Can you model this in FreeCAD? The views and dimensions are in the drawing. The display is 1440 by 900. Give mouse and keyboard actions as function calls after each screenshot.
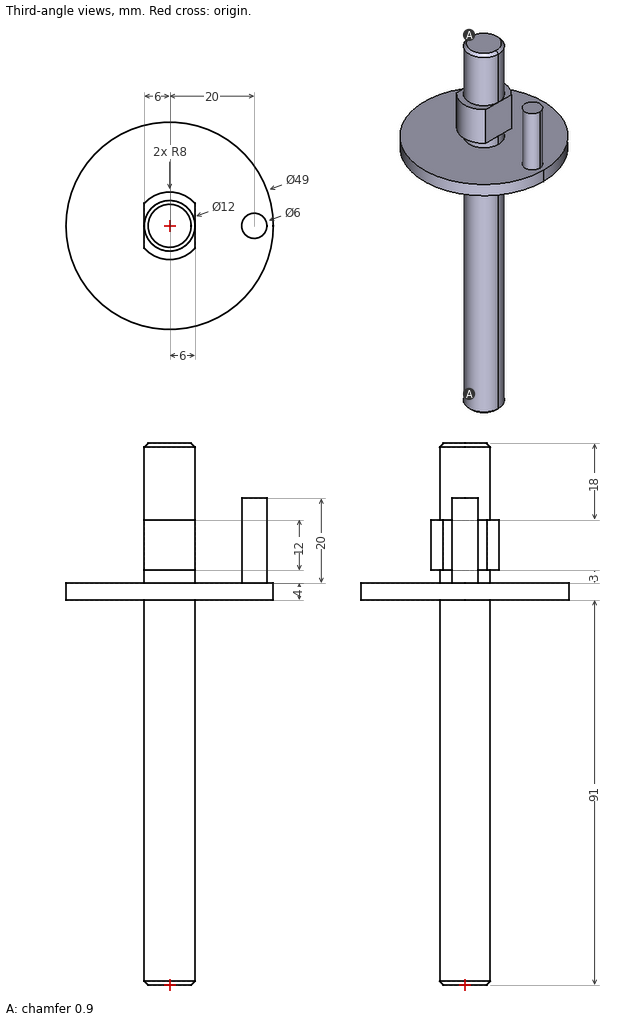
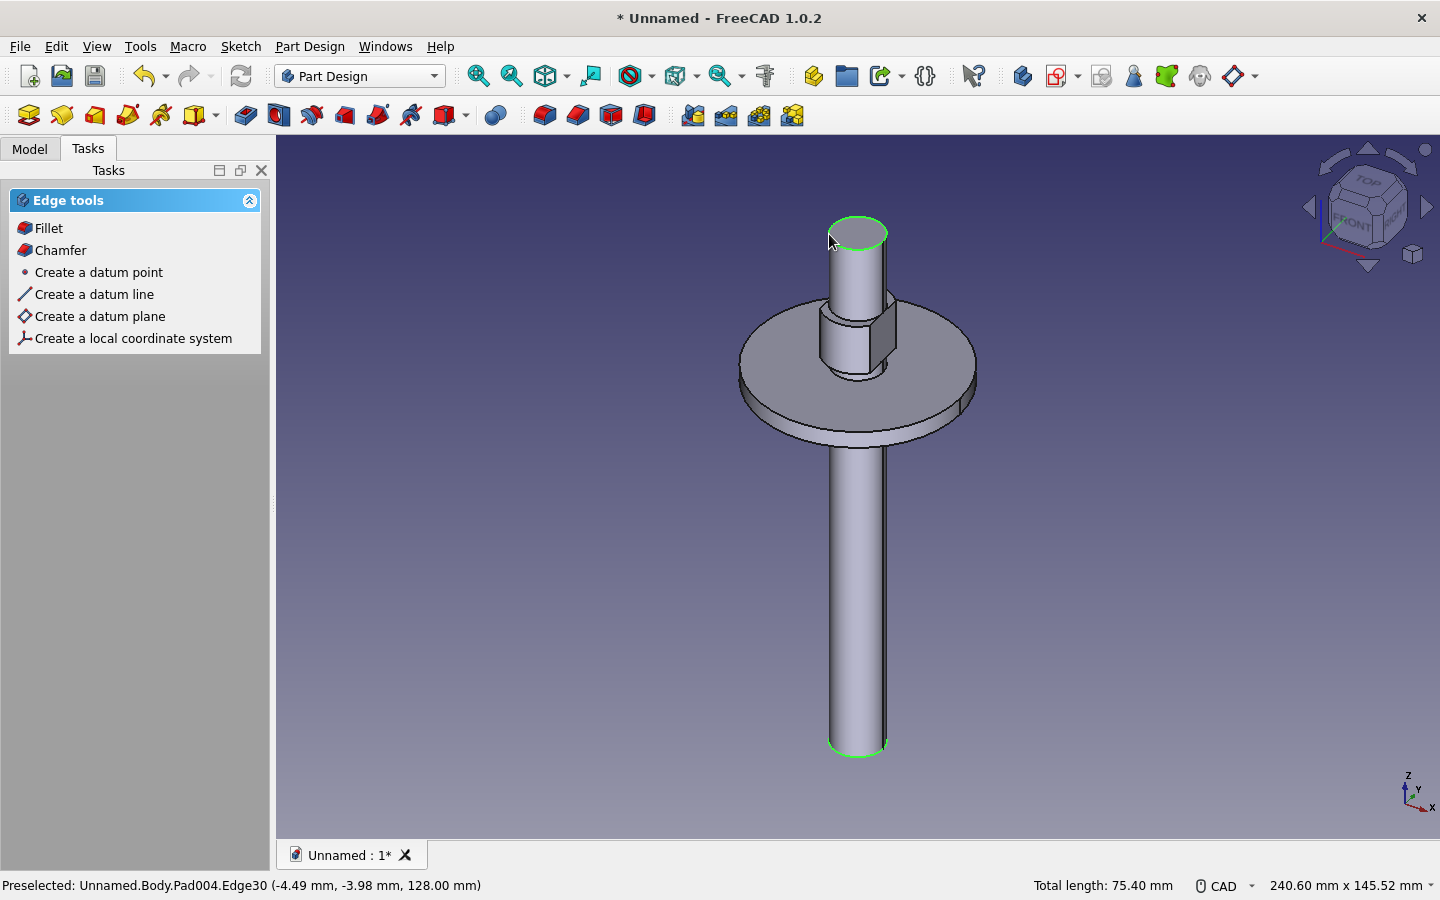
click(578, 116)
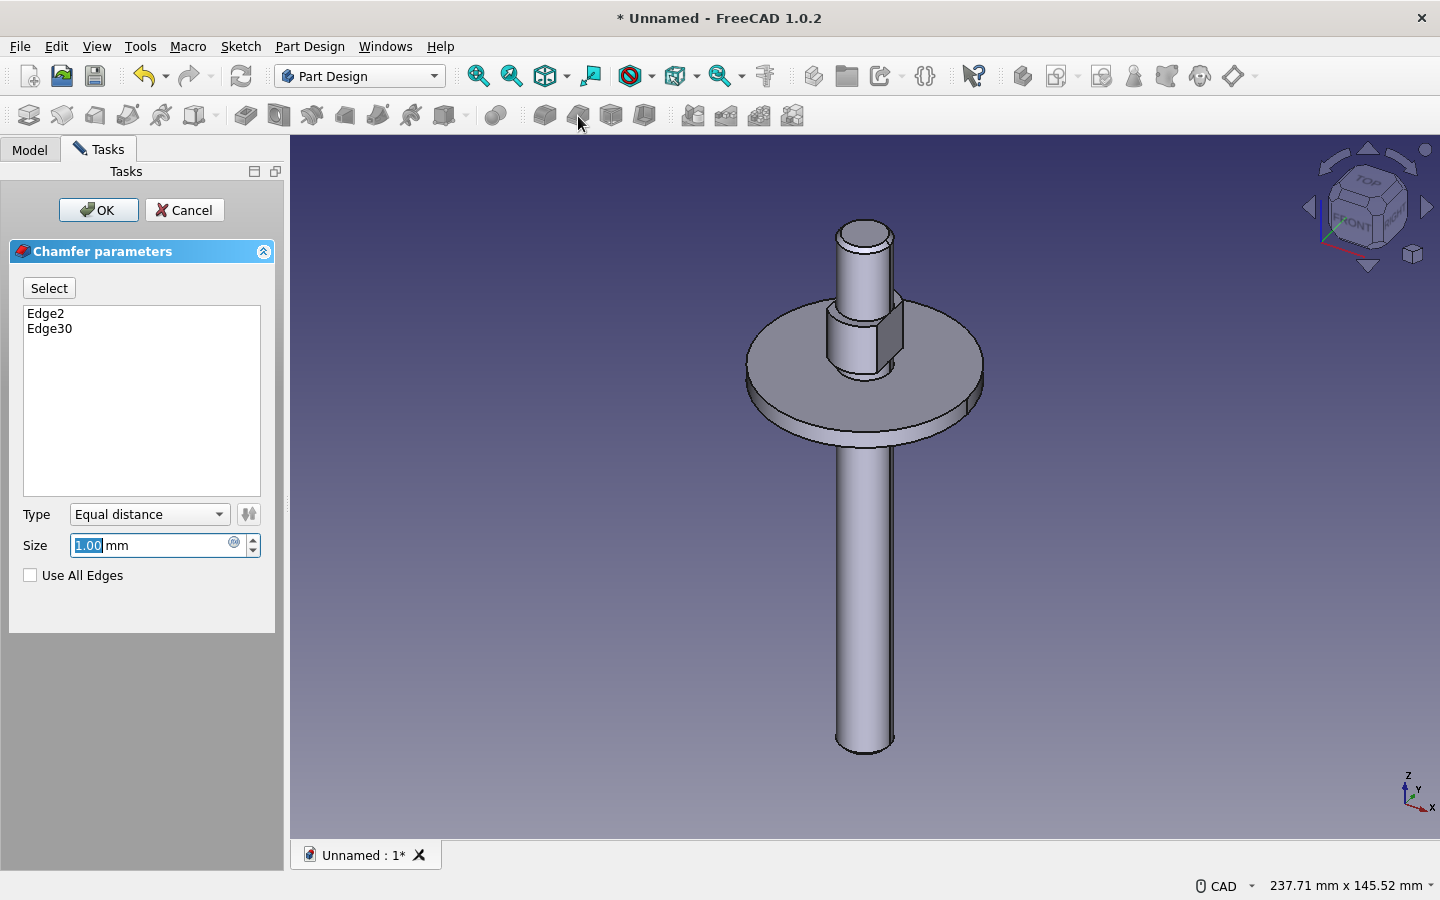
text(0.9)
key(Tab)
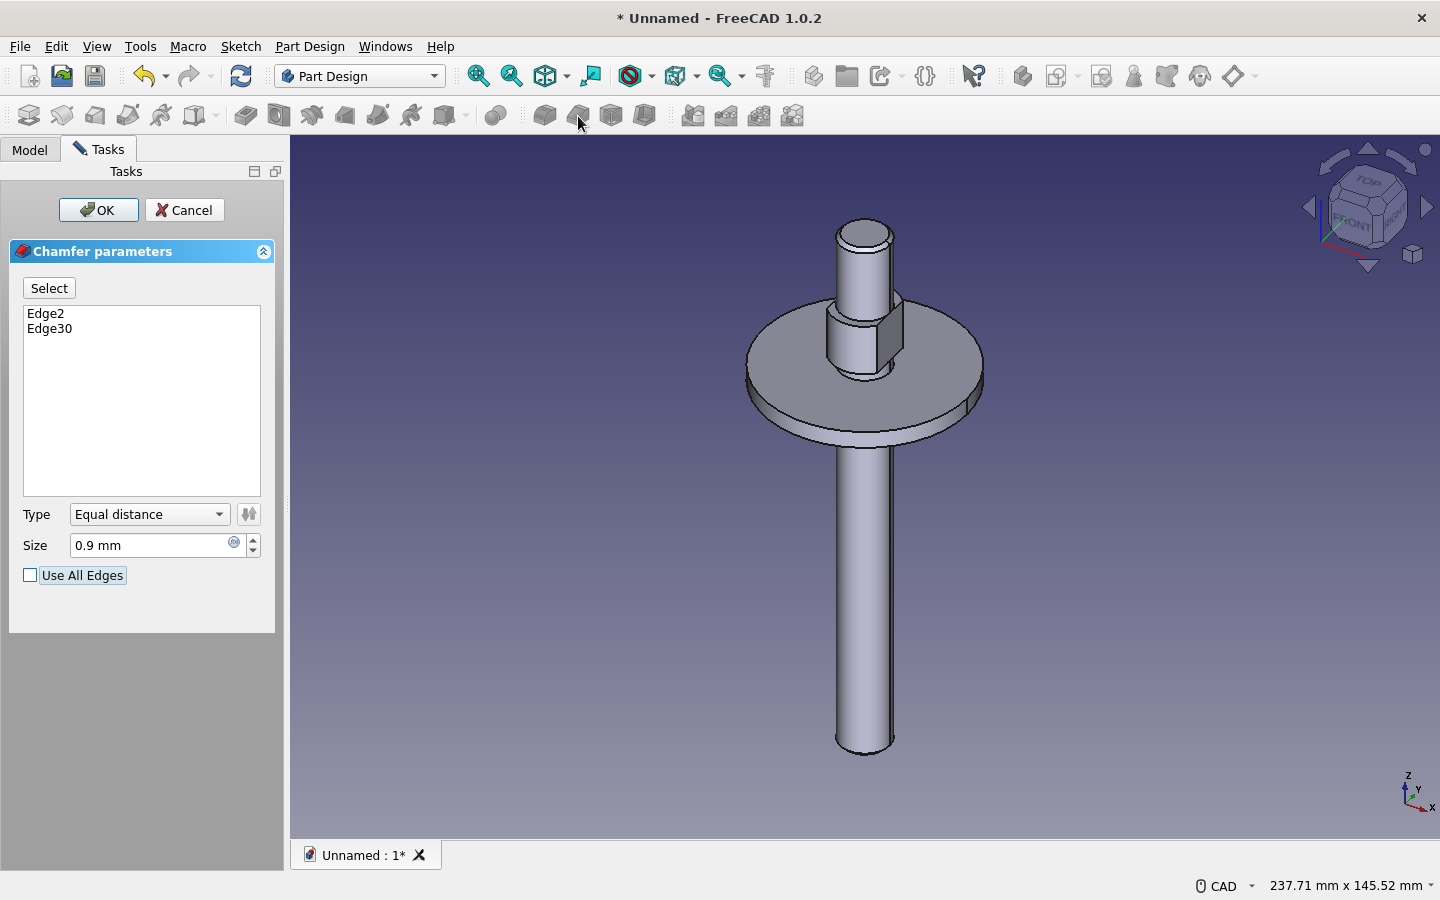
click(99, 210)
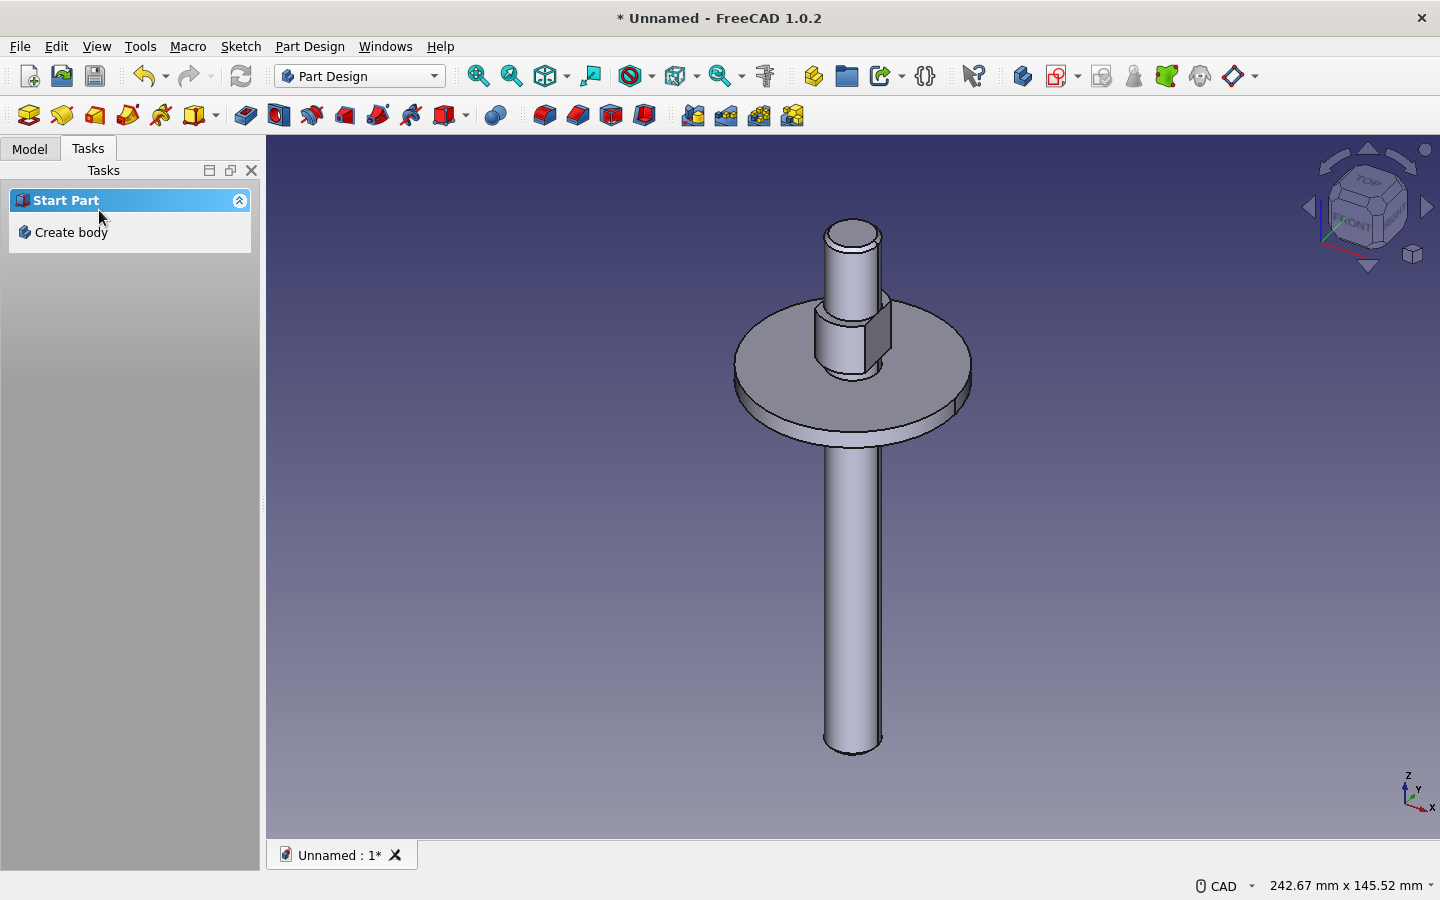
click(928, 366)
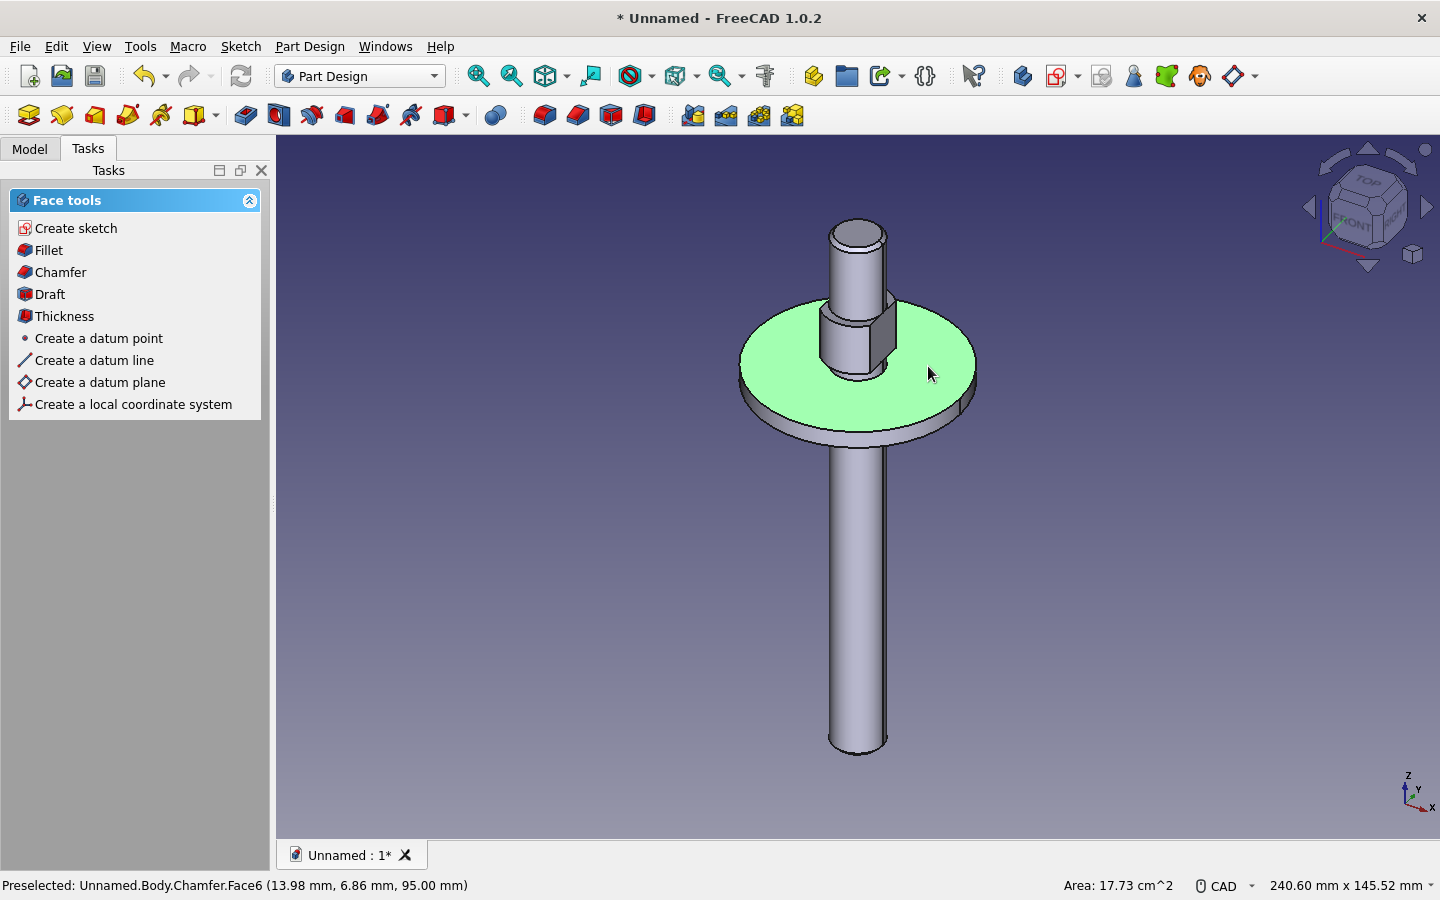
click(1056, 76)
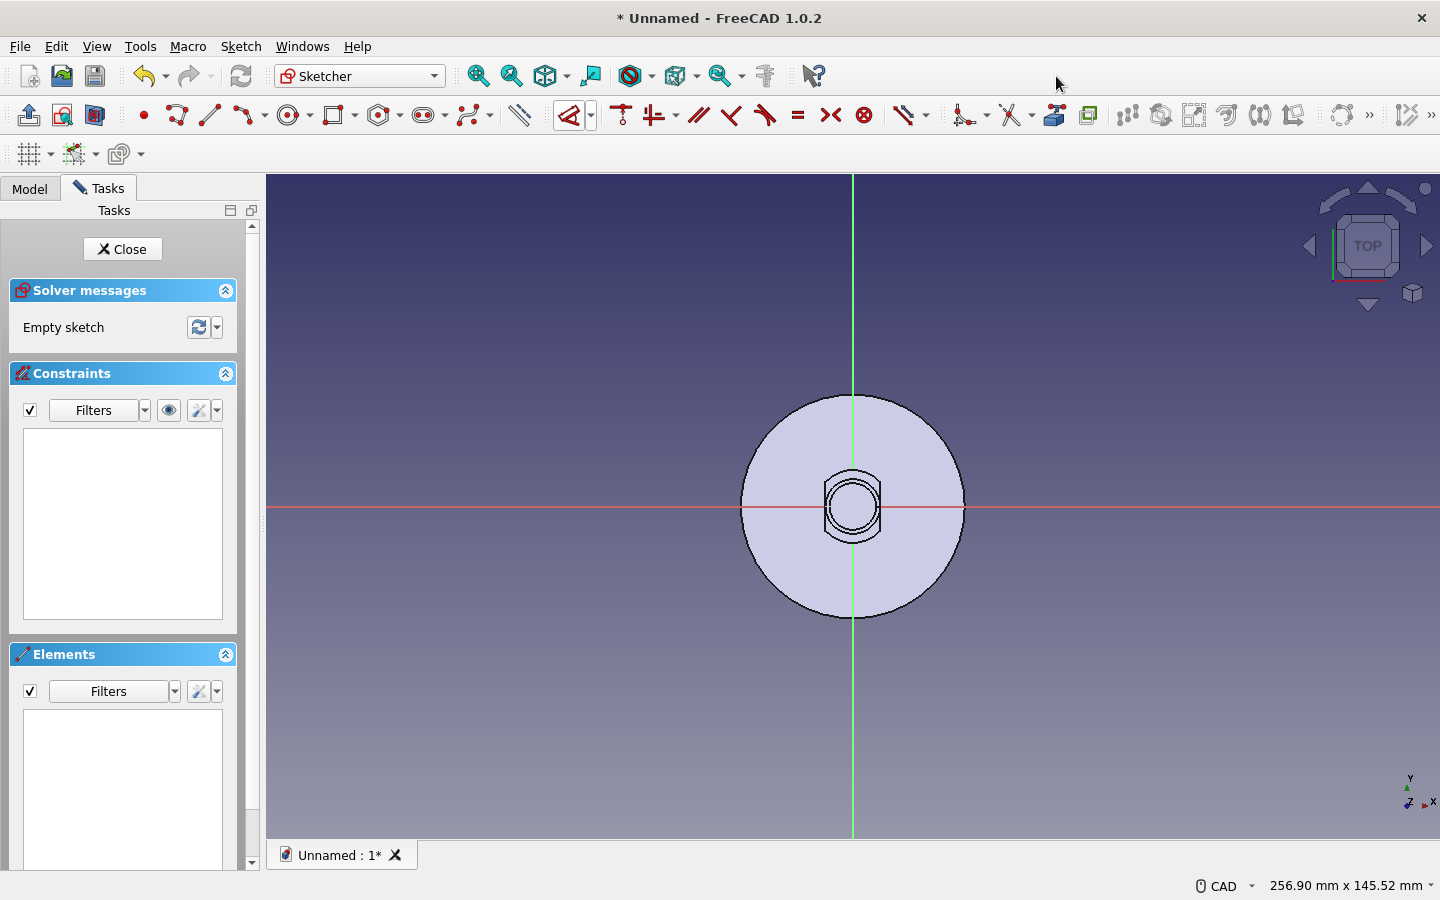
key(q)
key(s)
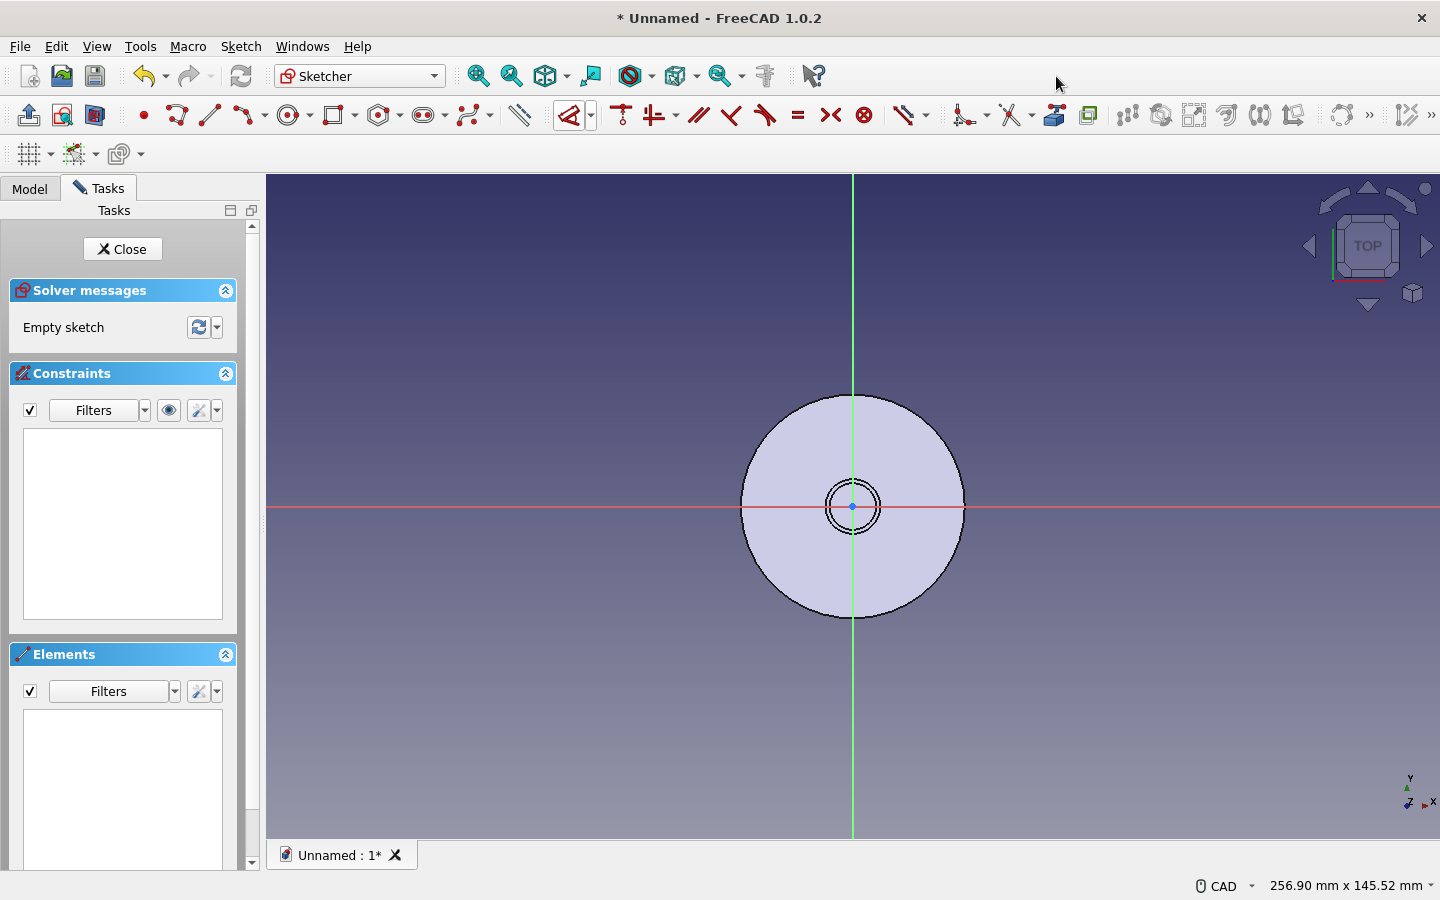
scroll(955, 506, up, 14)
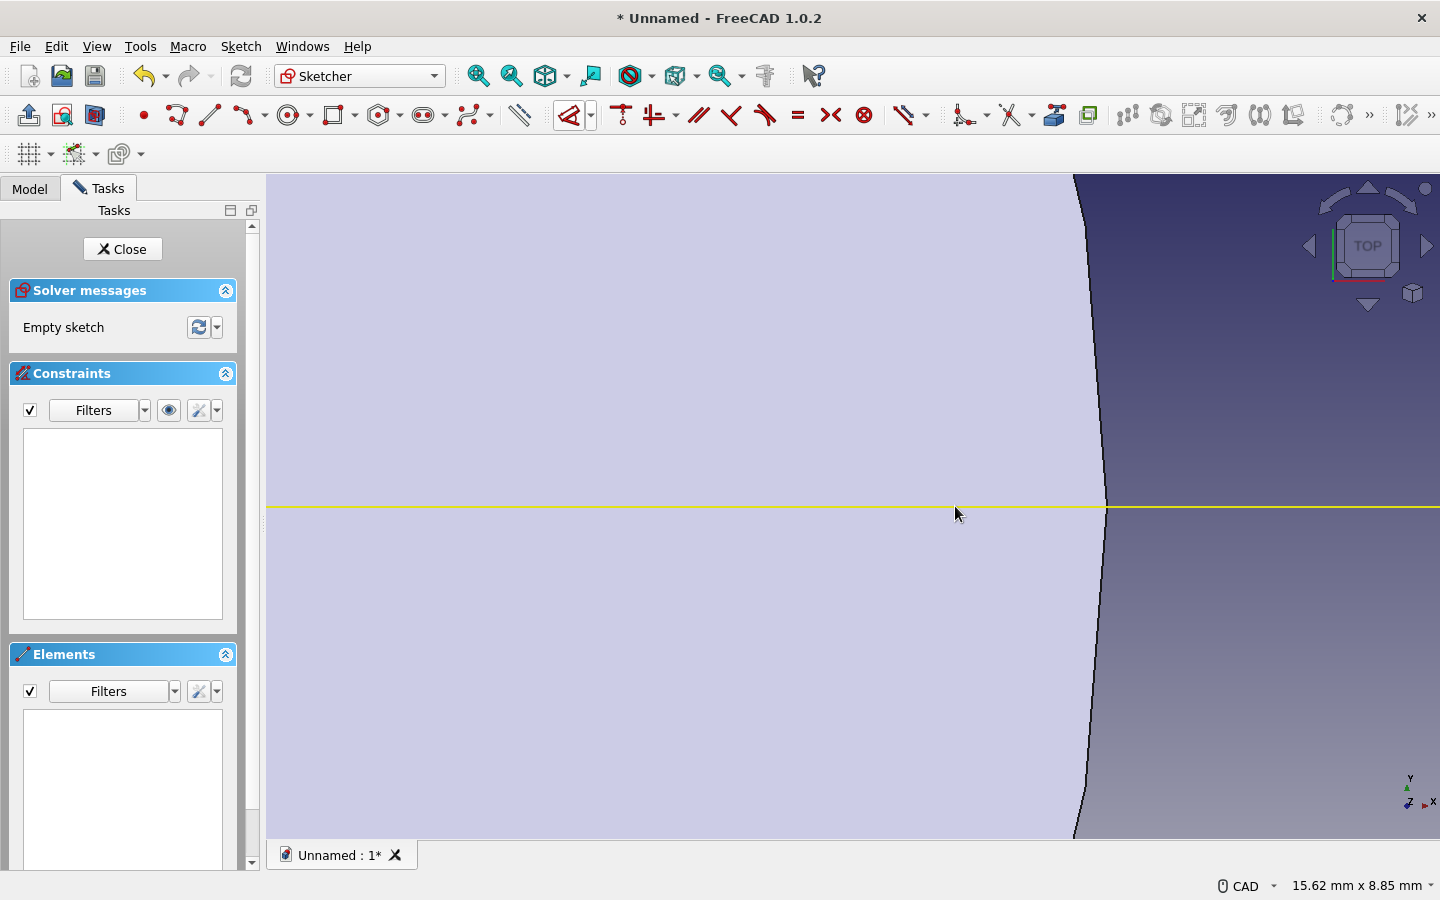
key(g)
key(c)